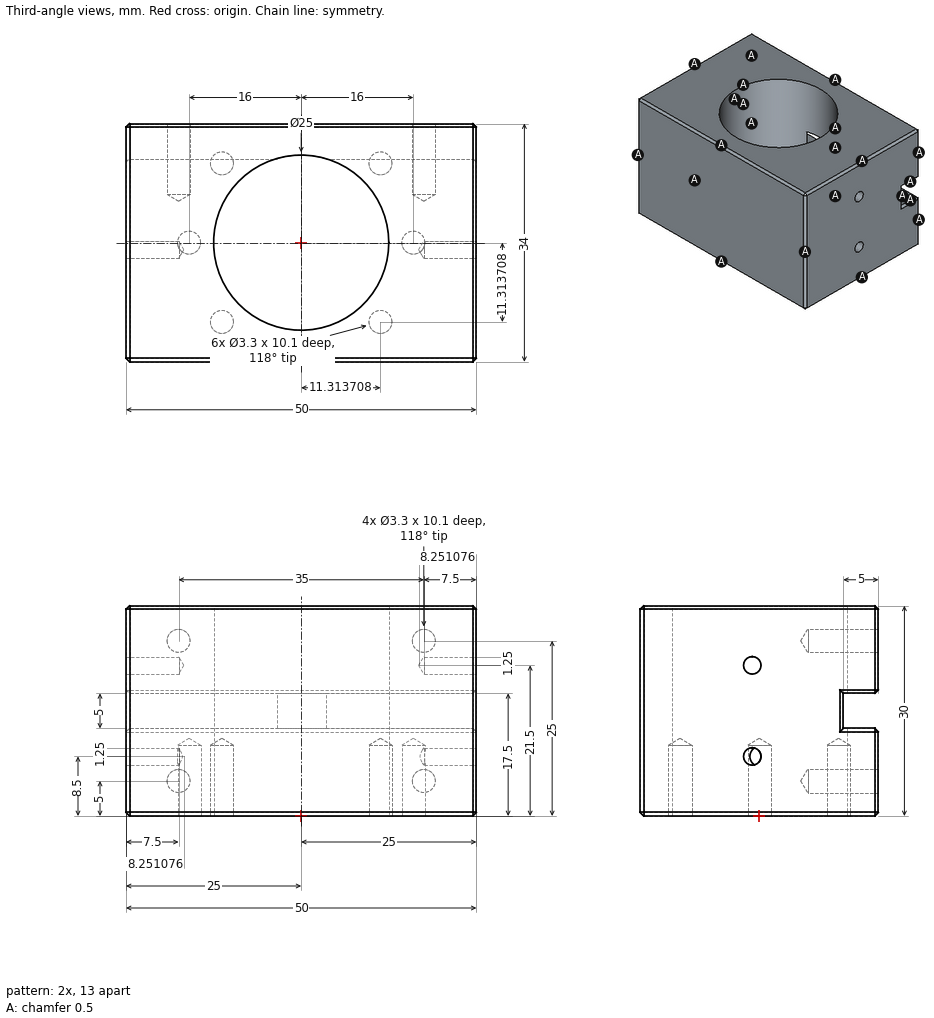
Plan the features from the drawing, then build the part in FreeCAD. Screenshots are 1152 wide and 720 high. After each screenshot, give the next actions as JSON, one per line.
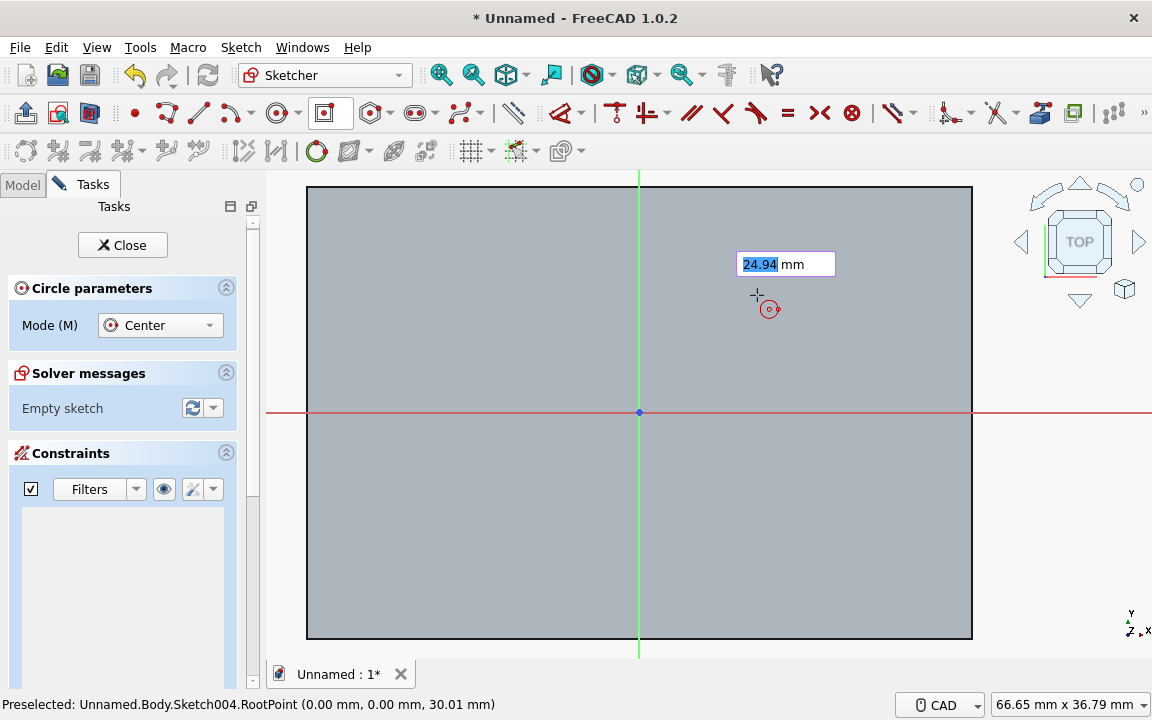
{"action": "type", "text": "25"}
{"action": "key", "text": "Return"}
{"action": "key", "text": "Escape"}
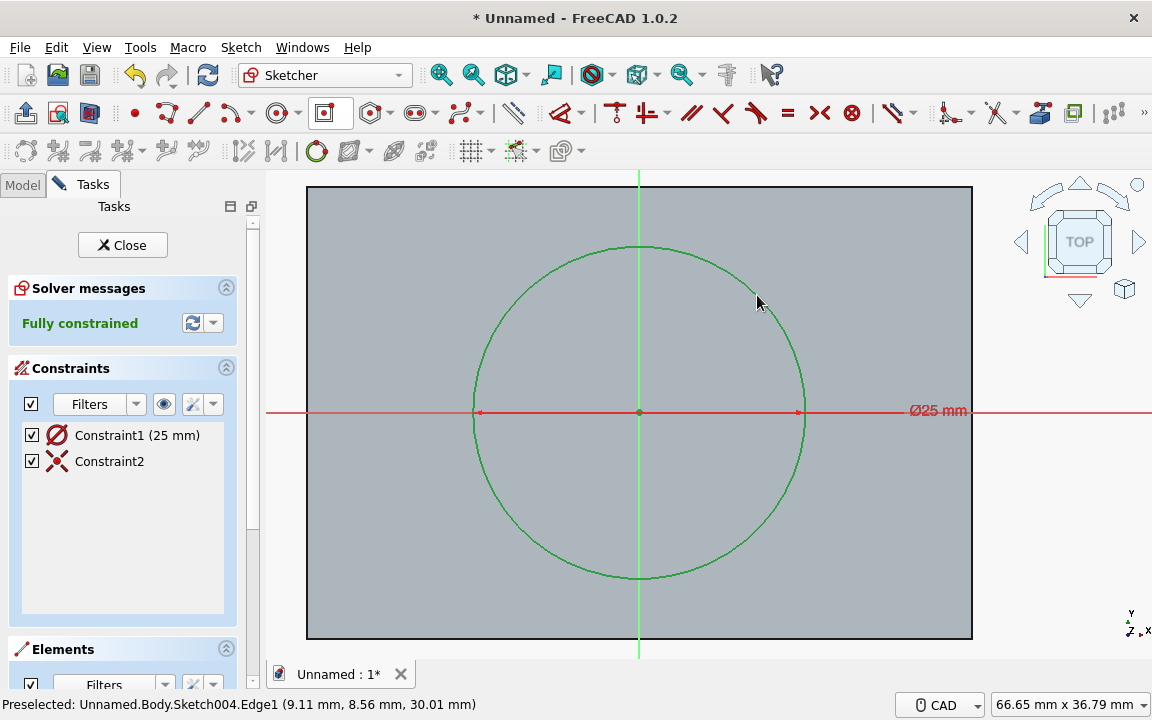
{"action": "left_click", "coordinate": [123, 245]}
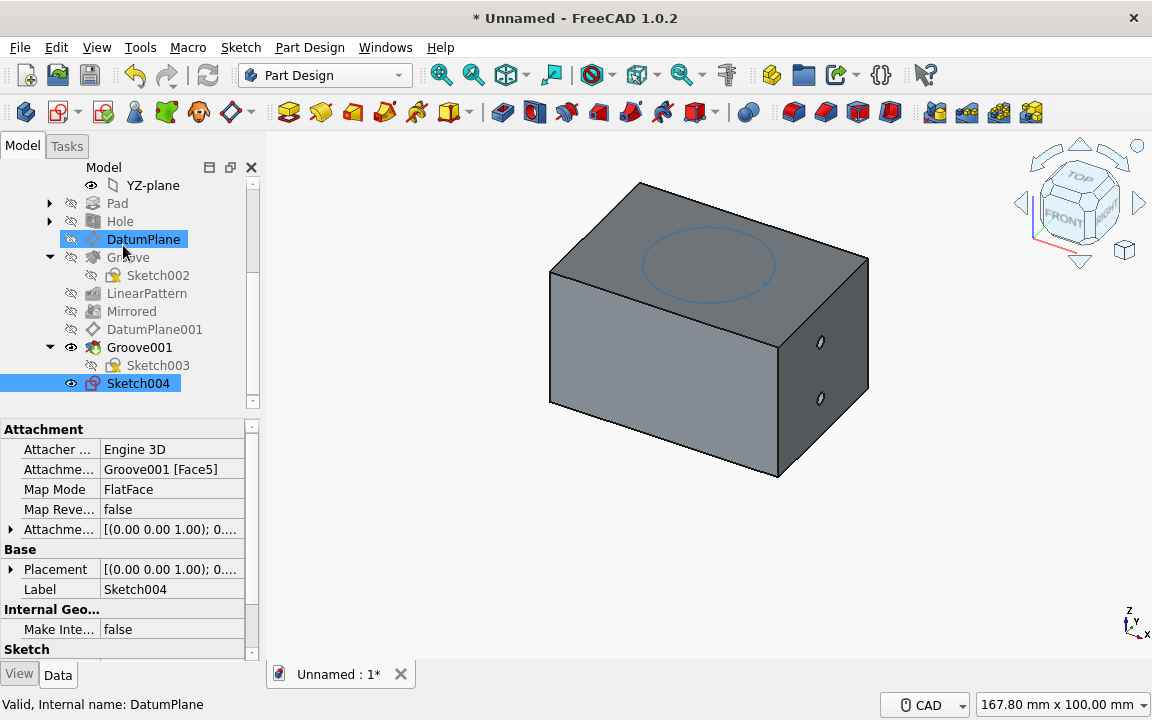
{"action": "left_click", "coordinate": [504, 112]}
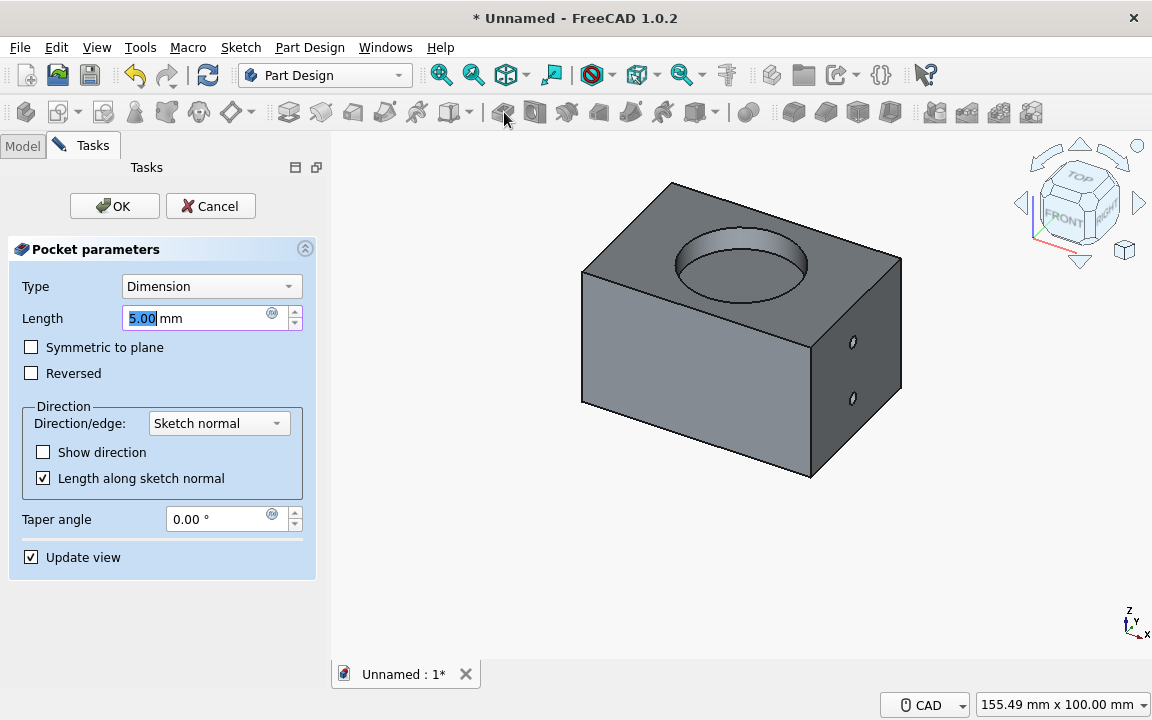
{"action": "left_click", "coordinate": [212, 286]}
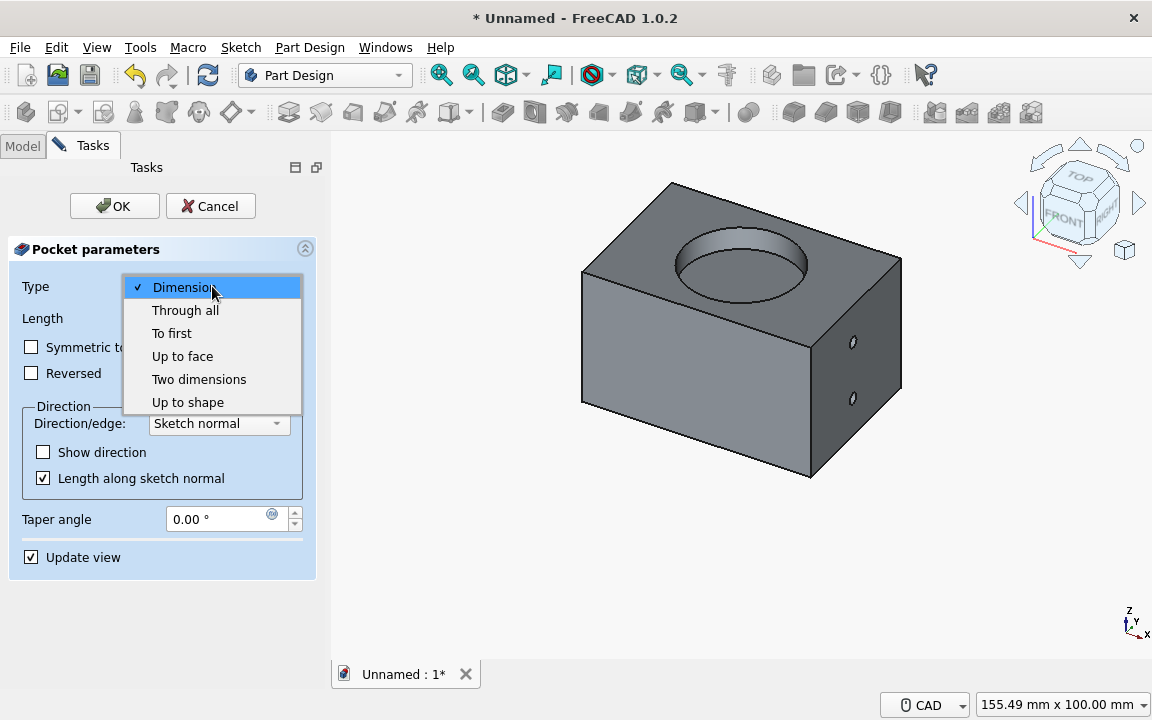
{"action": "left_click", "coordinate": [212, 310]}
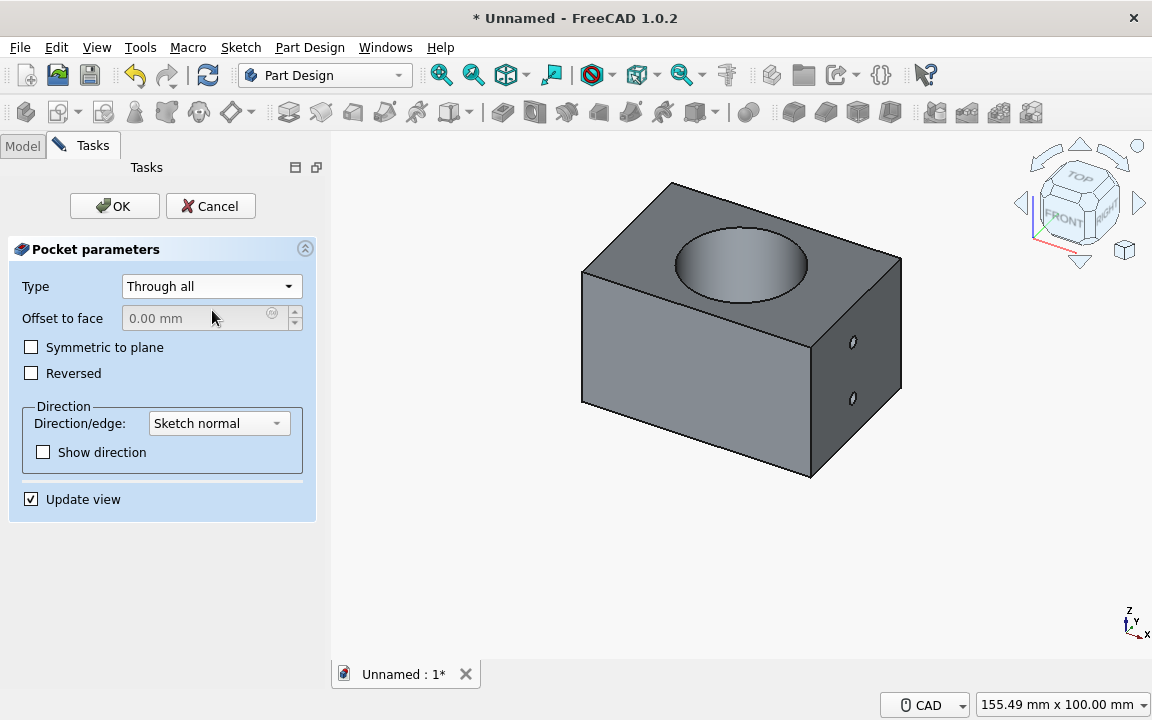
{"action": "left_click", "coordinate": [115, 206]}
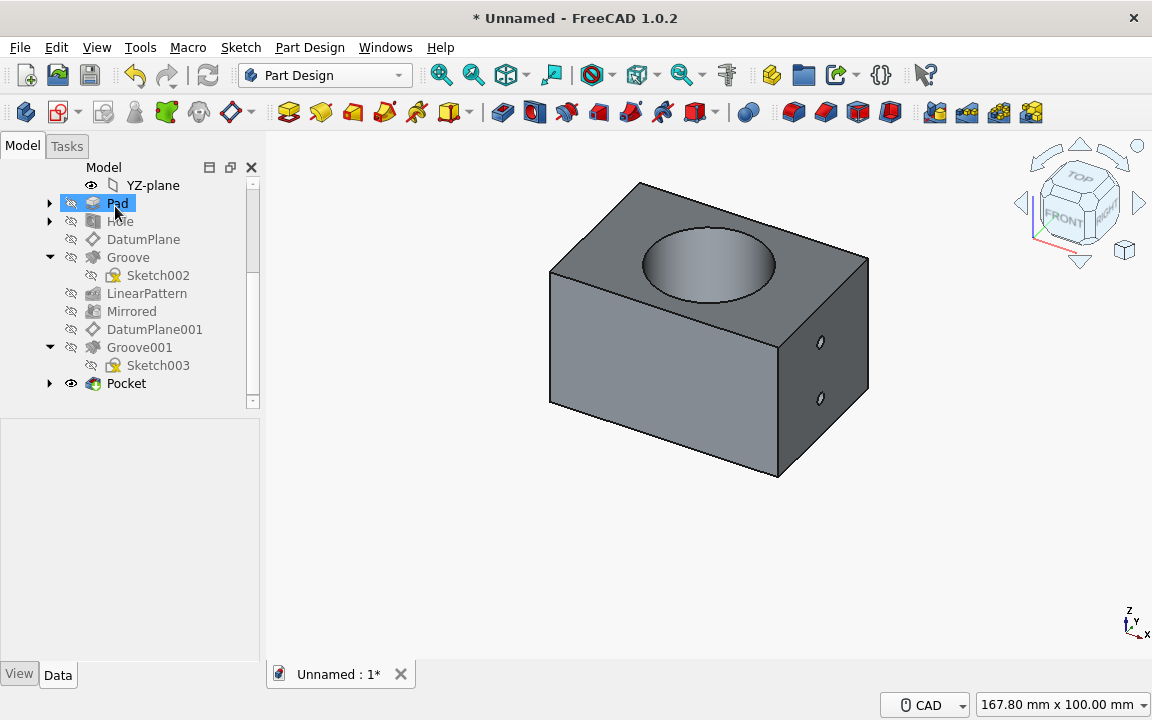
{"action": "key", "text": "4"}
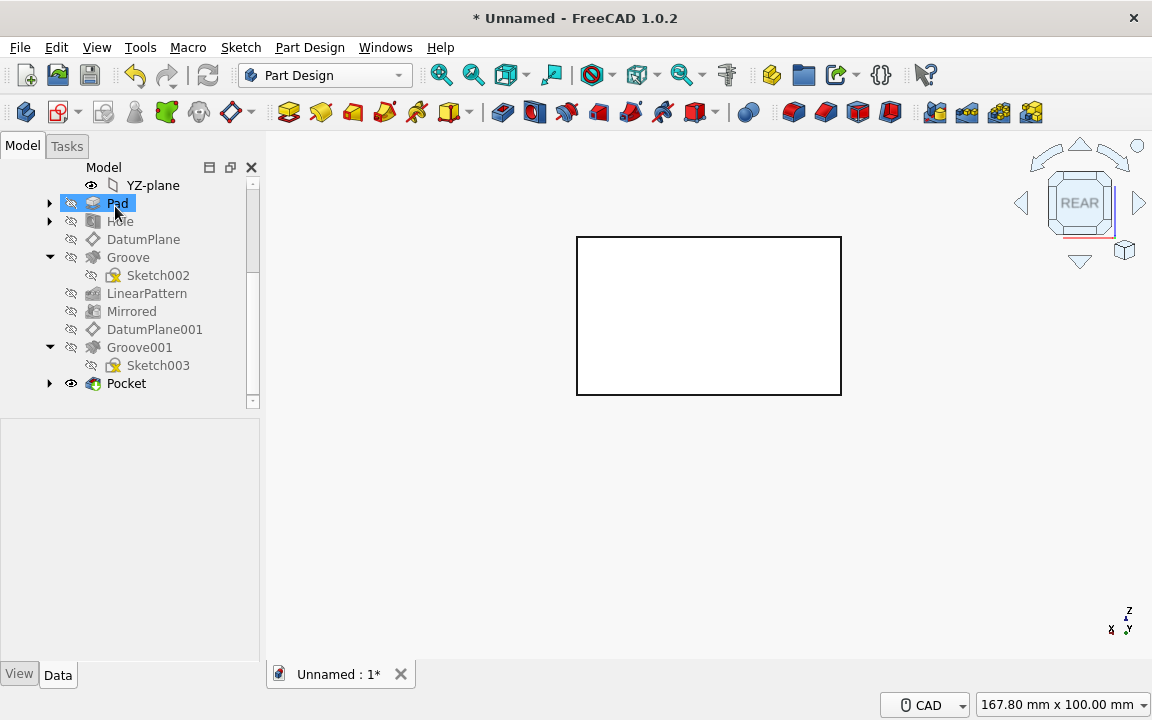
{"action": "key", "text": "v f"}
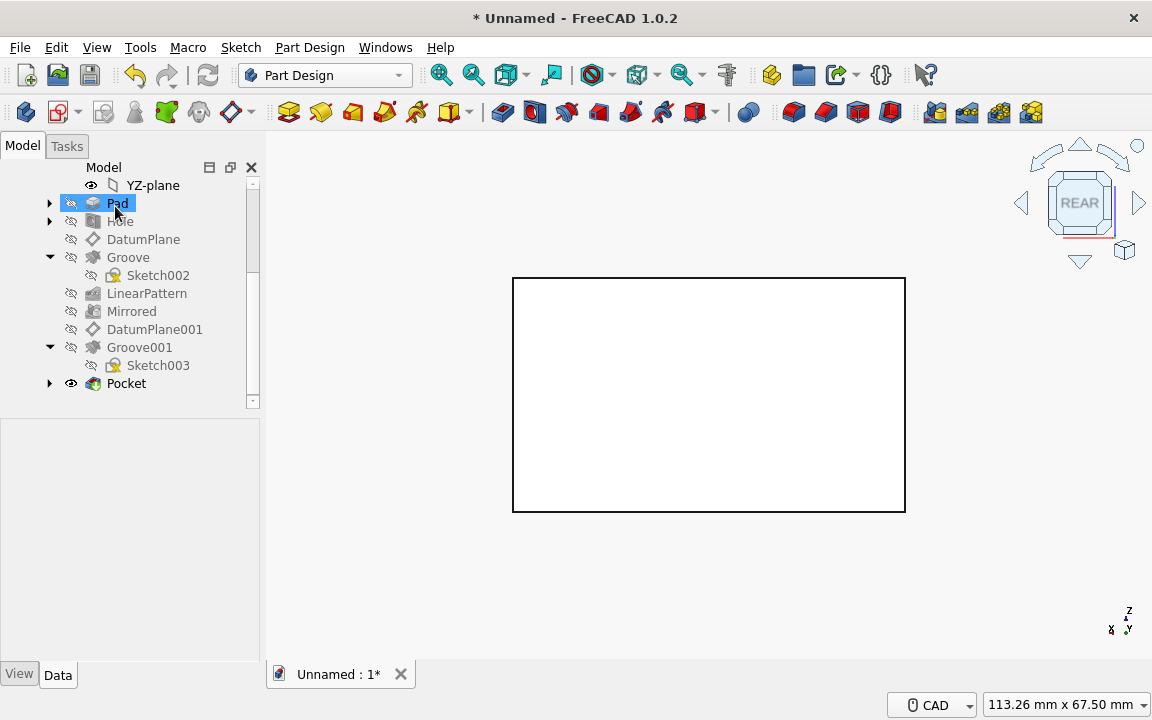
{"action": "left_click", "coordinate": [653, 394]}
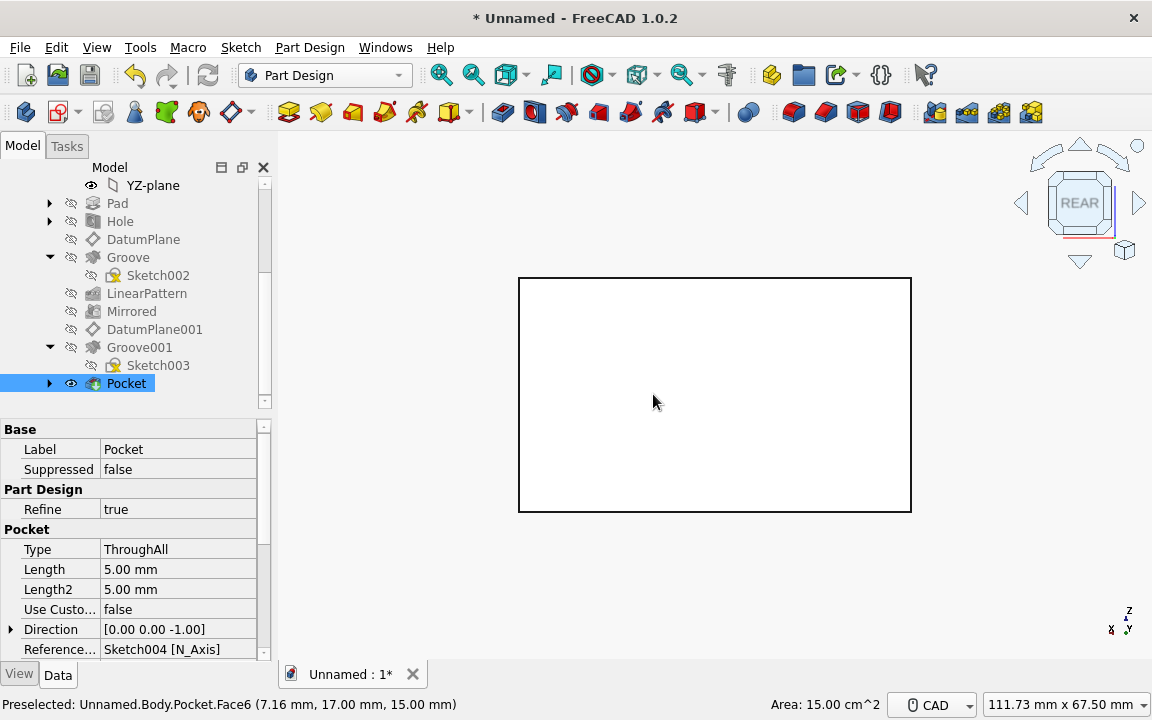
{"action": "left_click", "coordinate": [58, 112]}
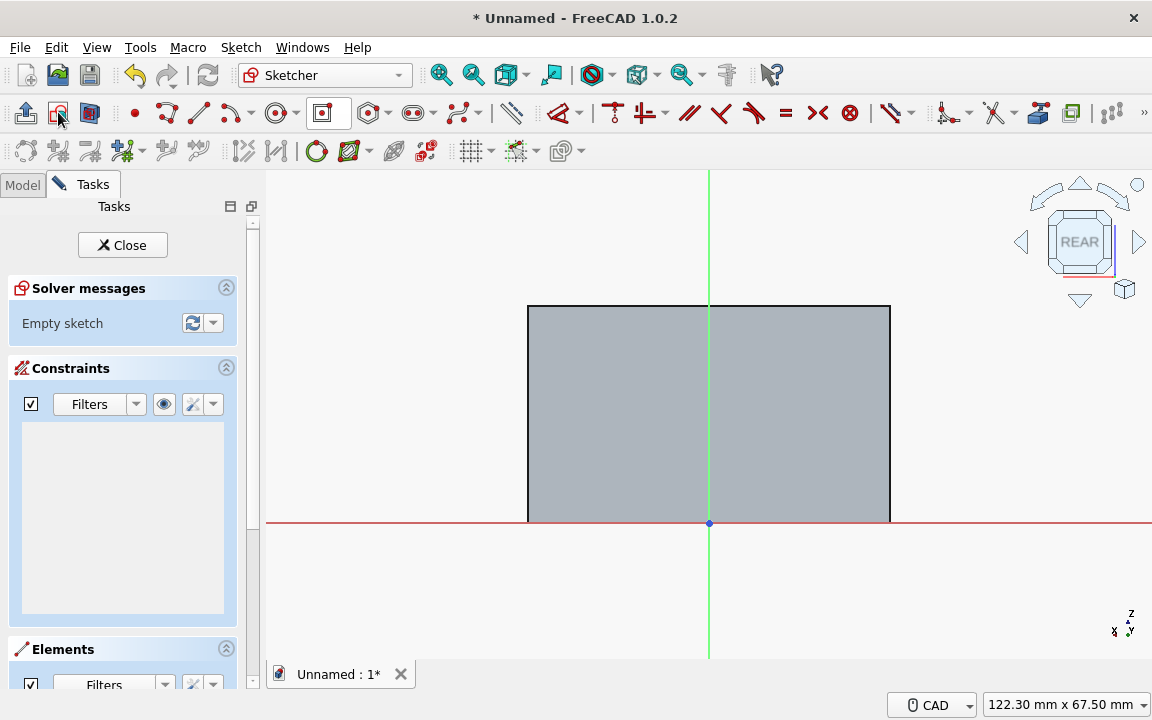
{"action": "scroll", "coordinate": [848, 451], "scroll_direction": "up", "scroll_amount": 2}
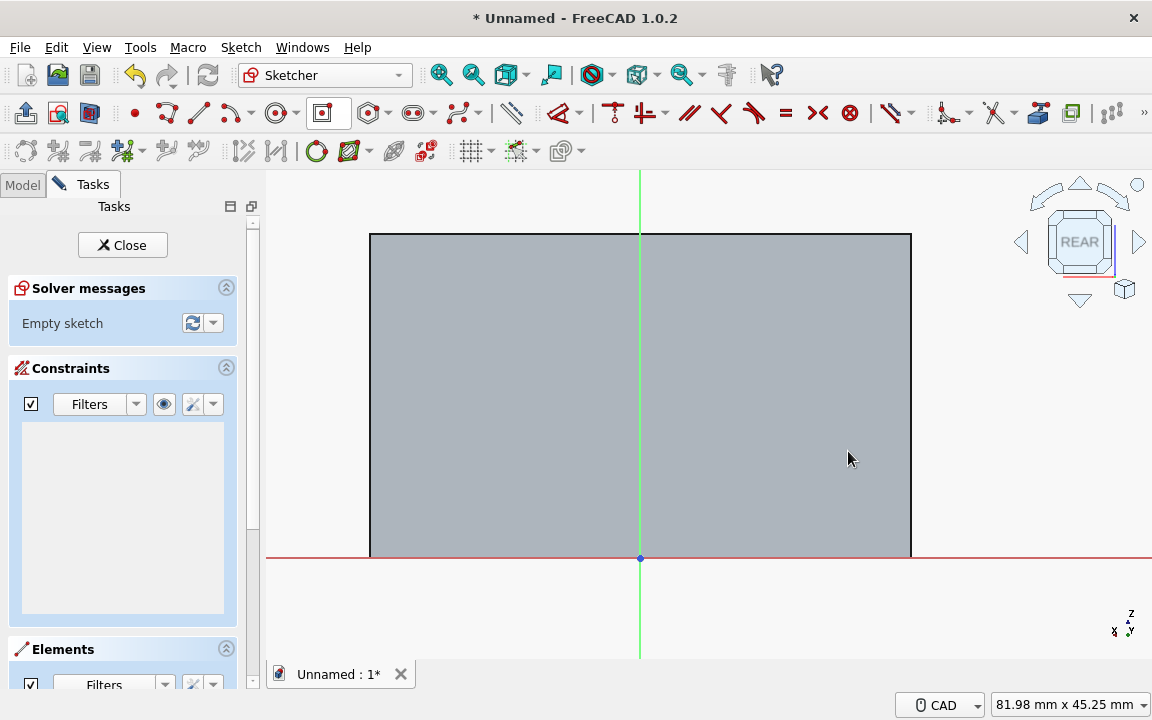
{"action": "key", "text": "g c"}